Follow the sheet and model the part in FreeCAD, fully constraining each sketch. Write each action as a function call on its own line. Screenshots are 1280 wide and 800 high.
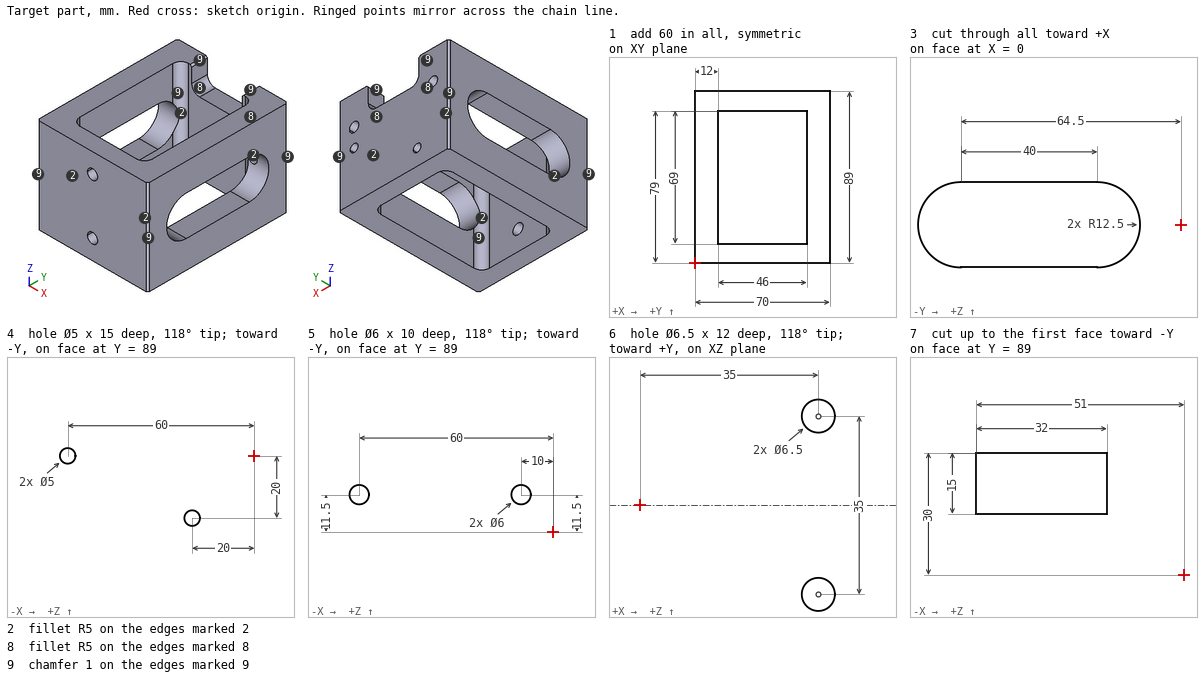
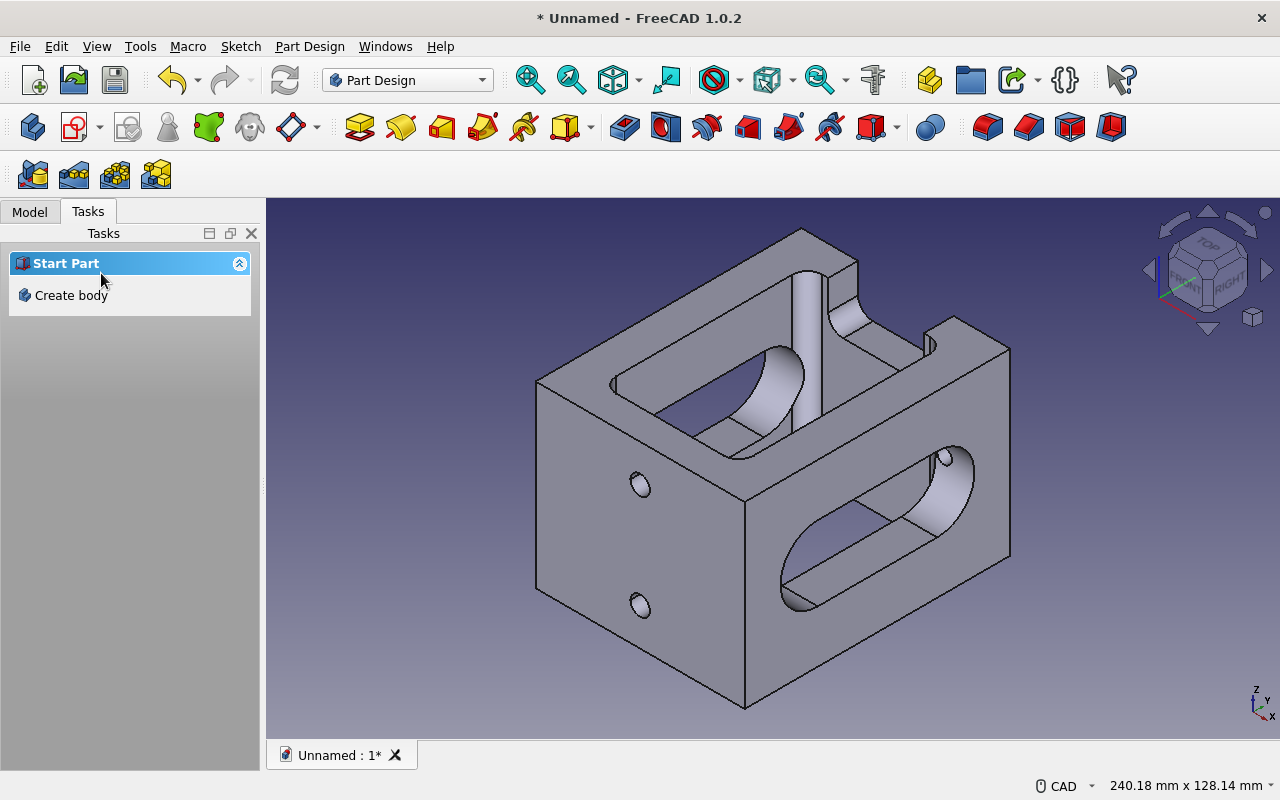
click(843, 268)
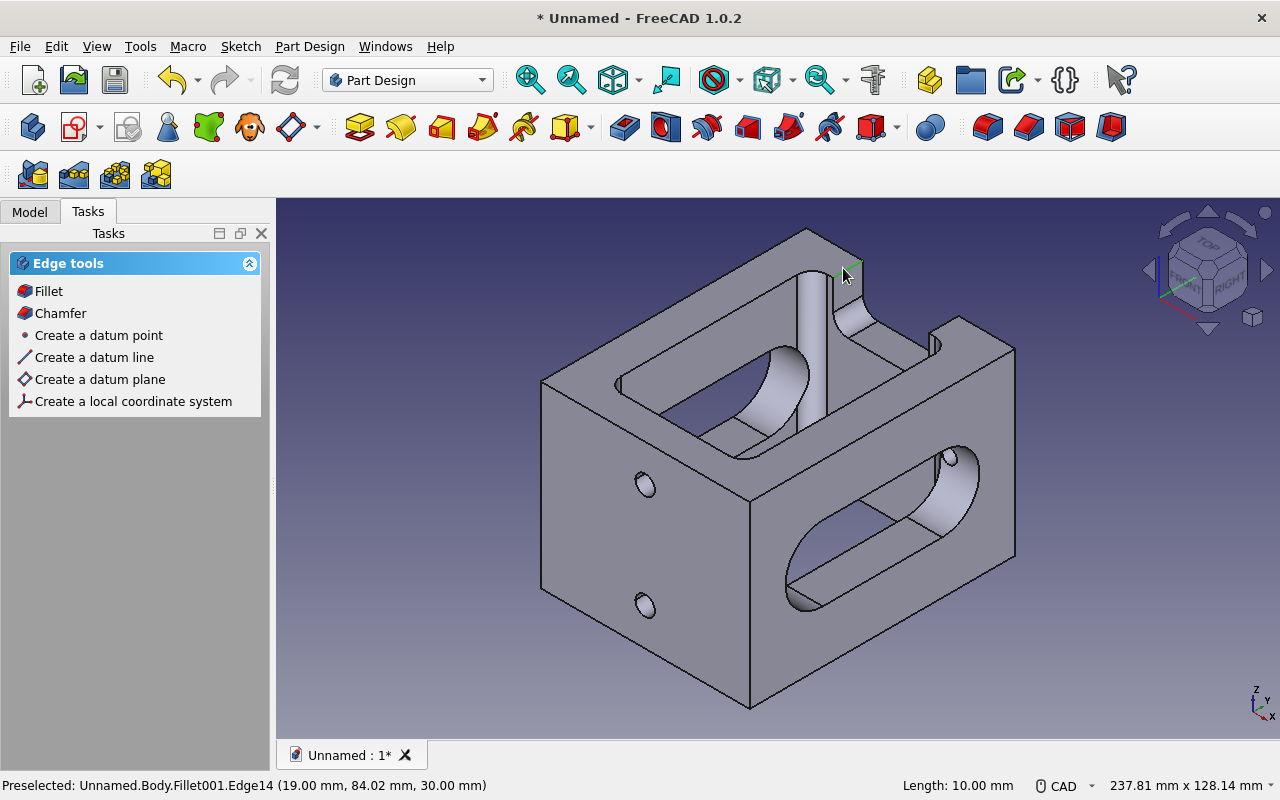
click(750, 605, ctrl)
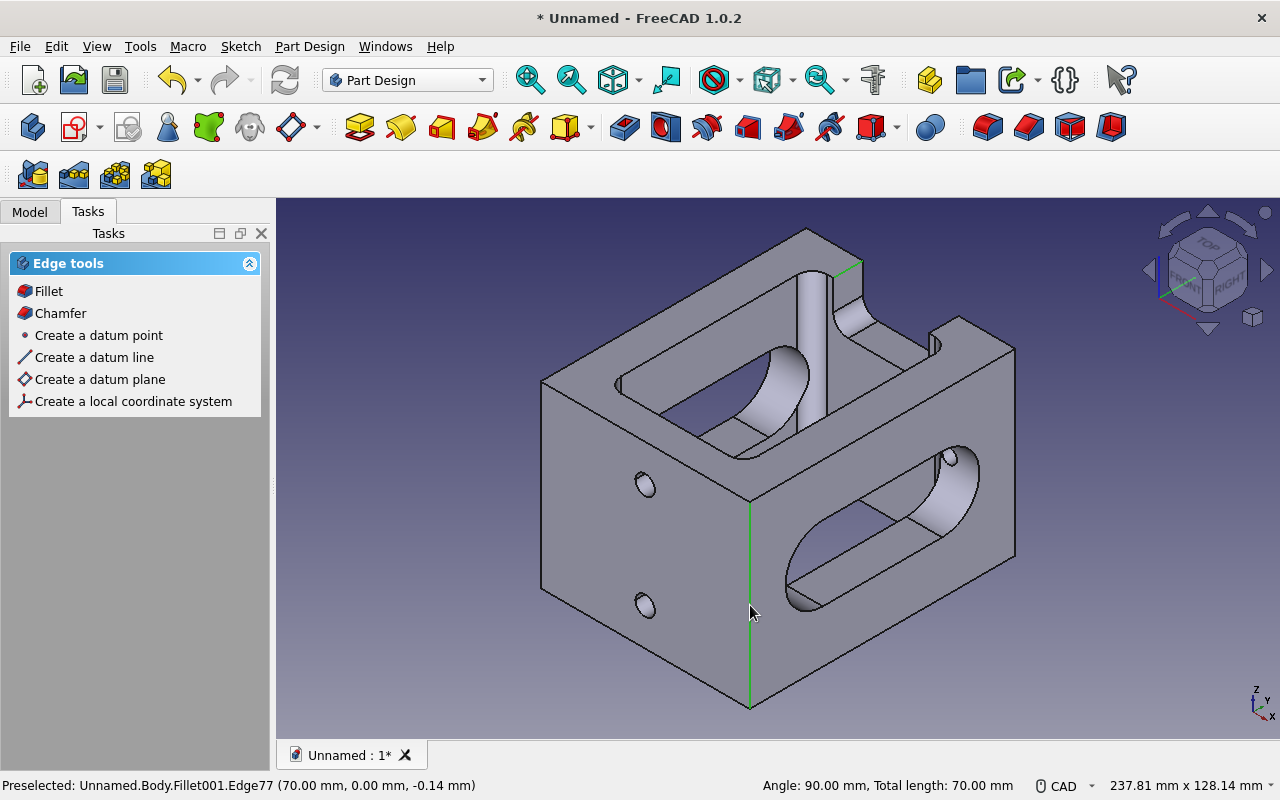
key(2)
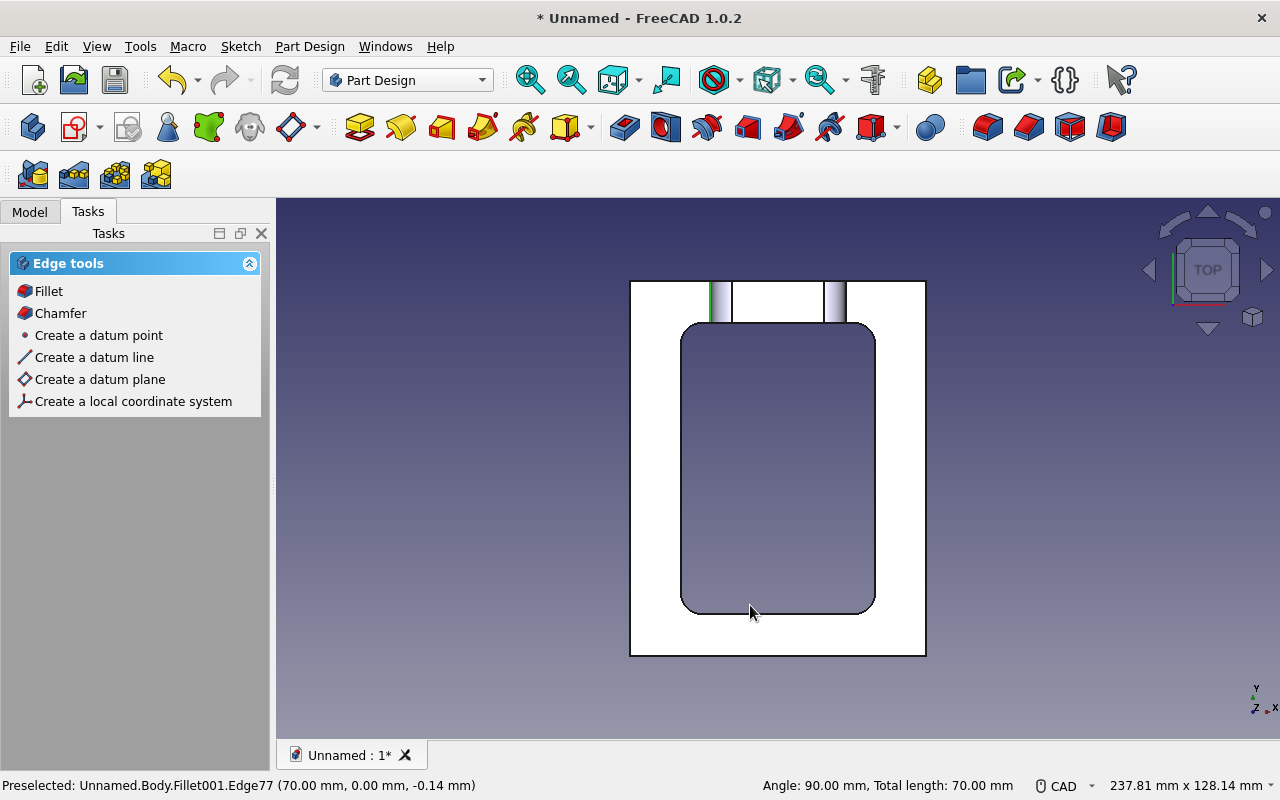
click(846, 301, ctrl)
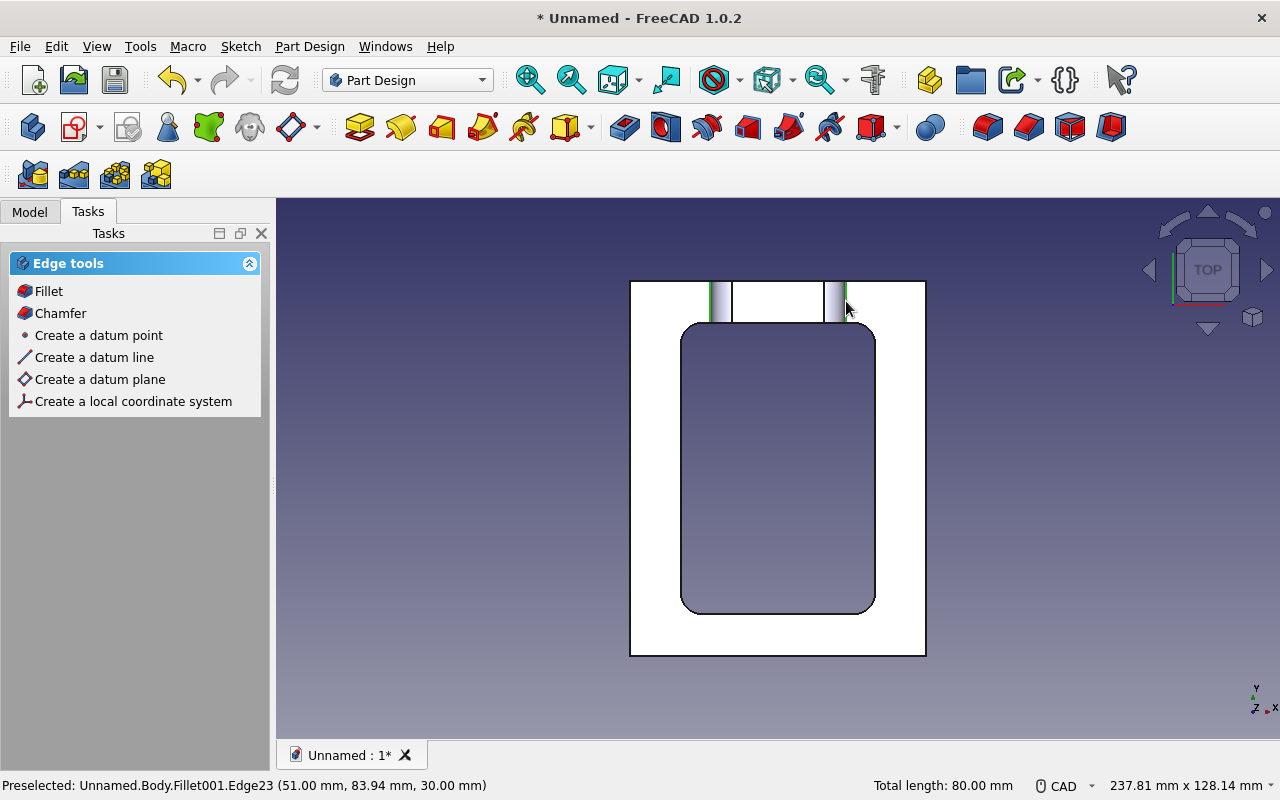
key(0)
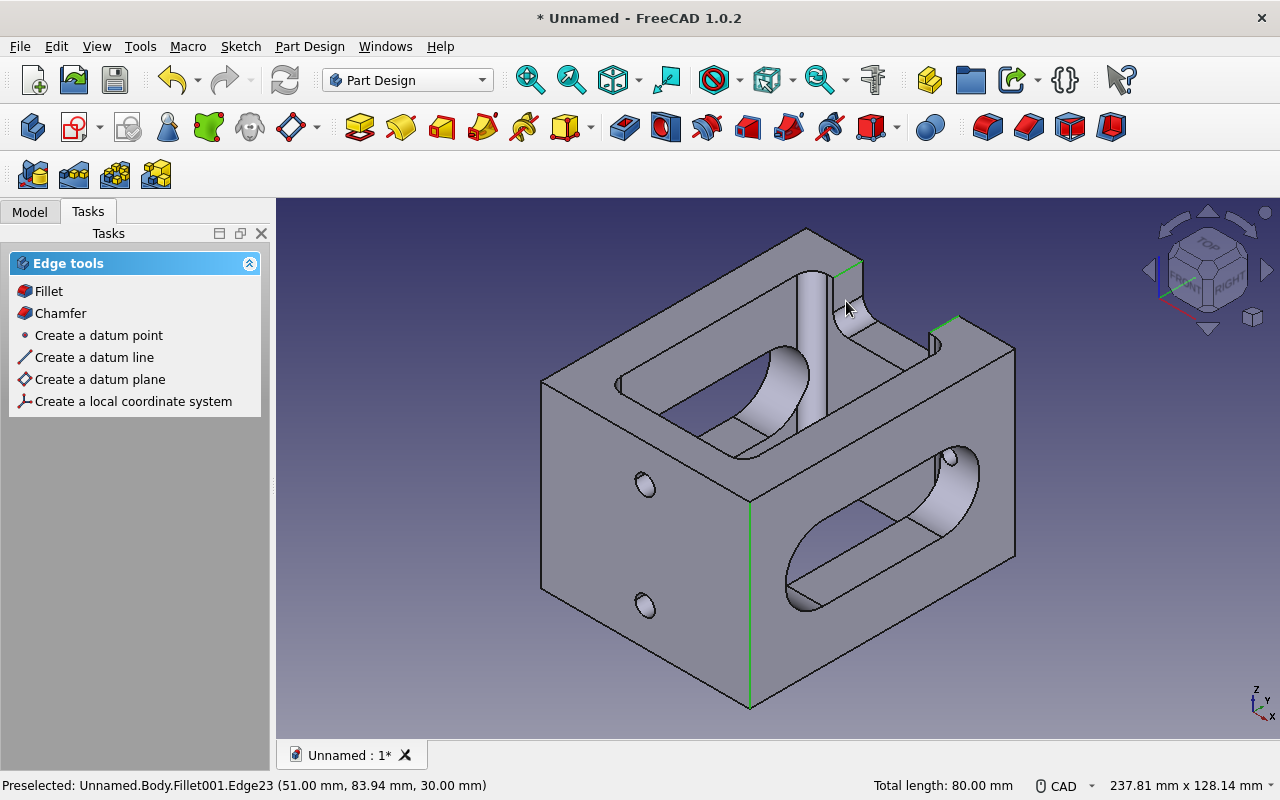
key(1)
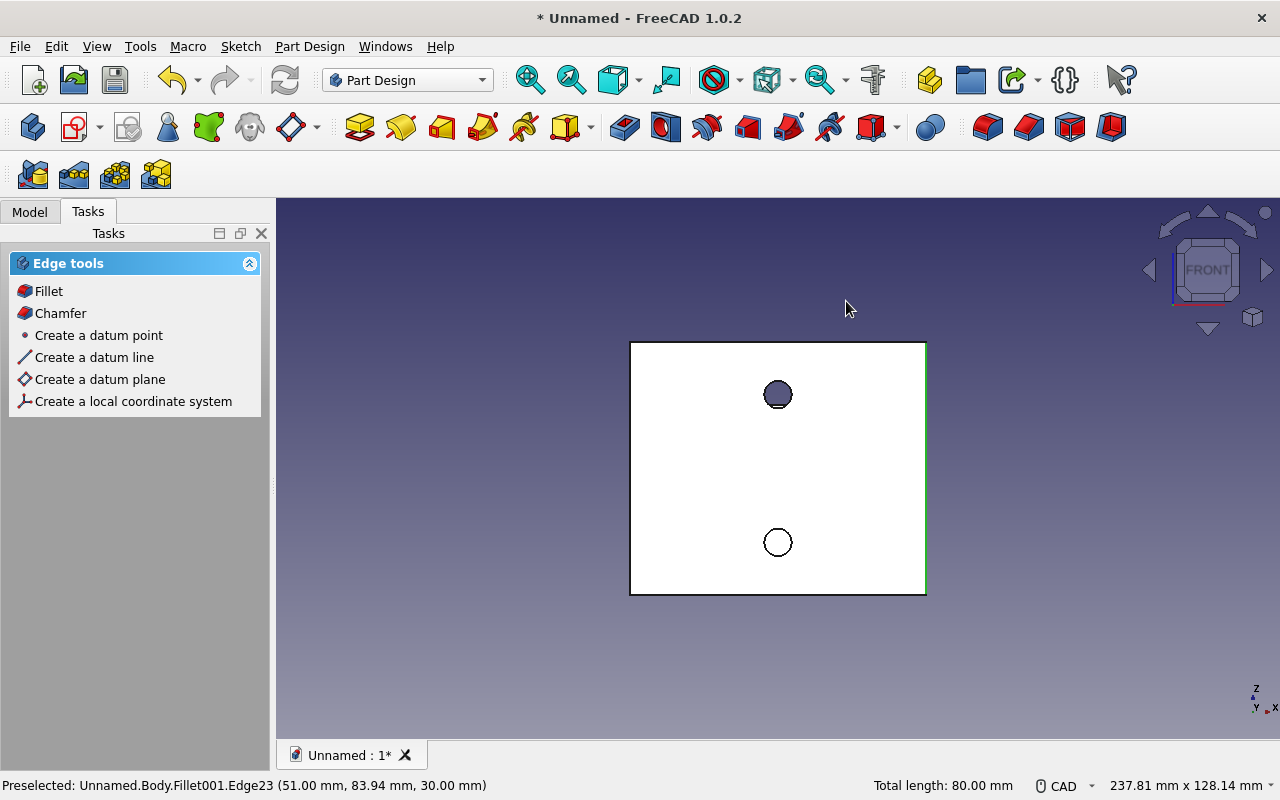
click(630, 468, ctrl)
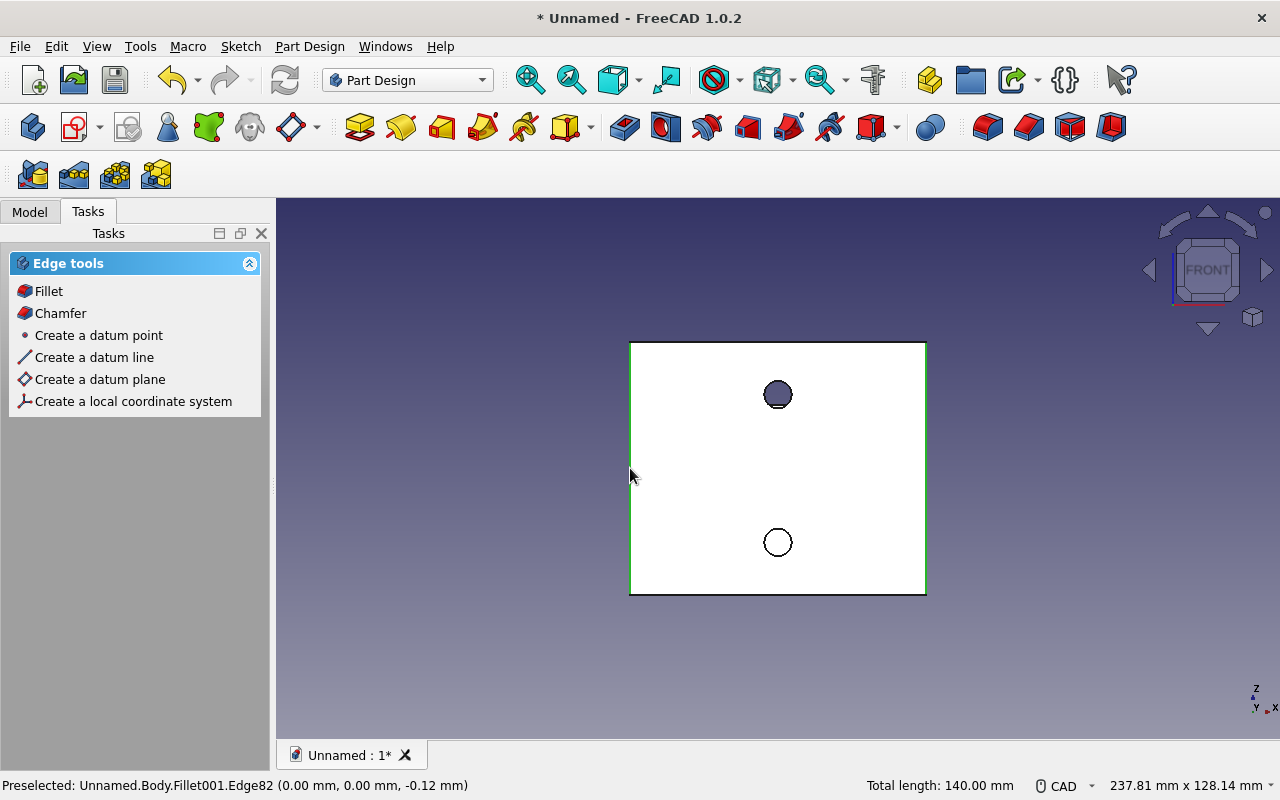
key(3)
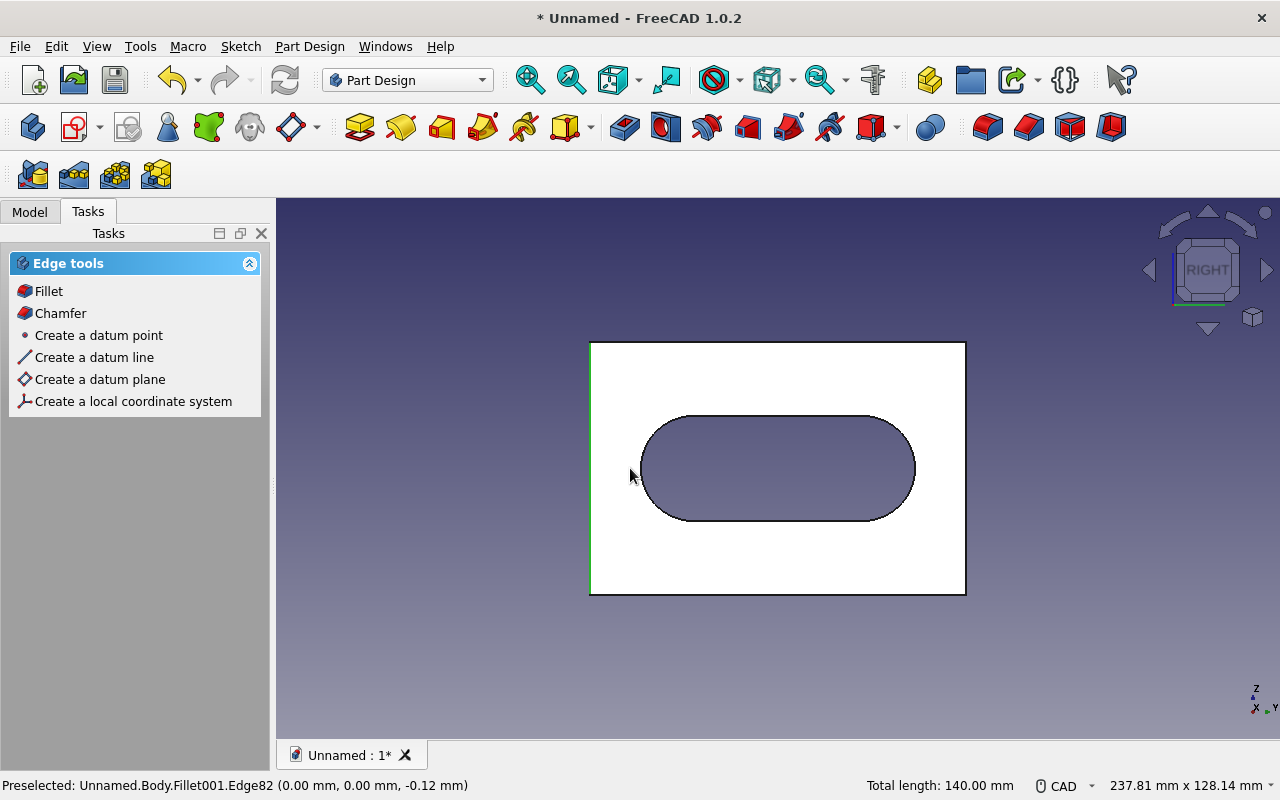
click(966, 468, ctrl)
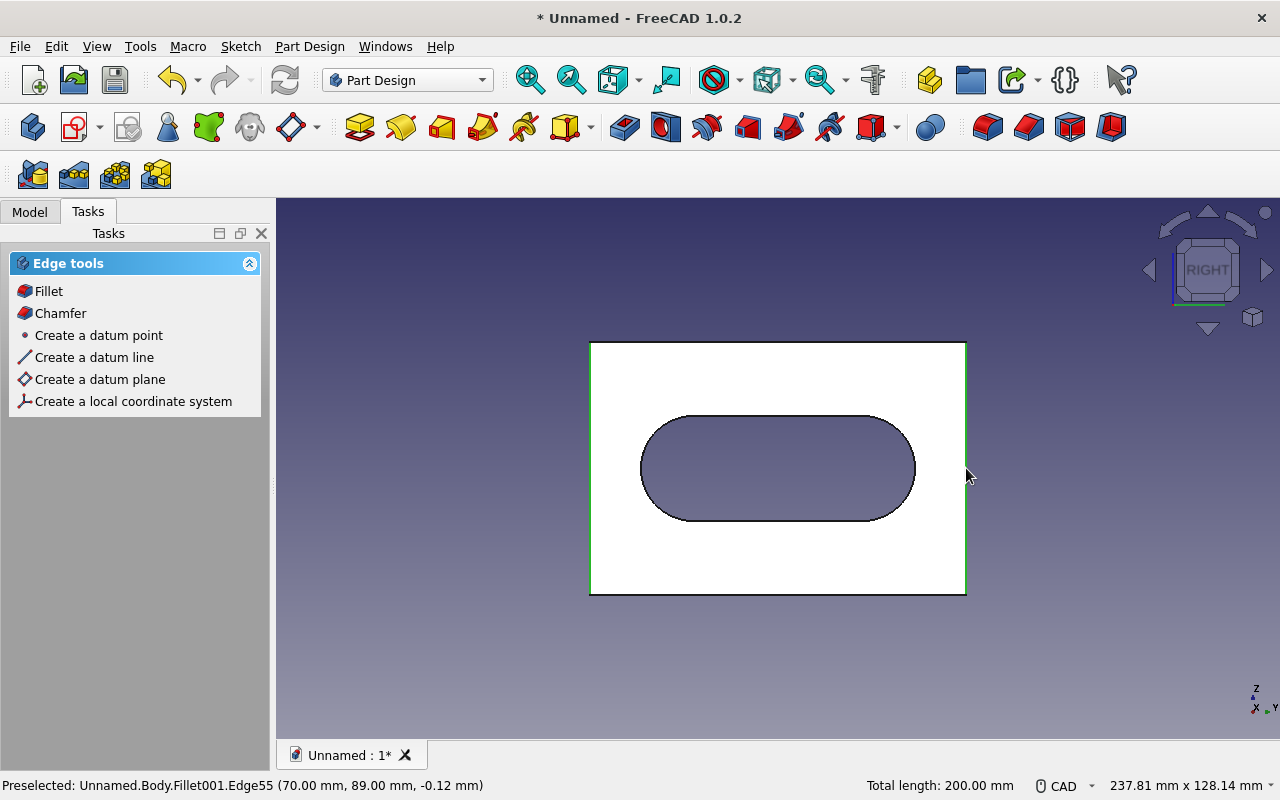
key(5)